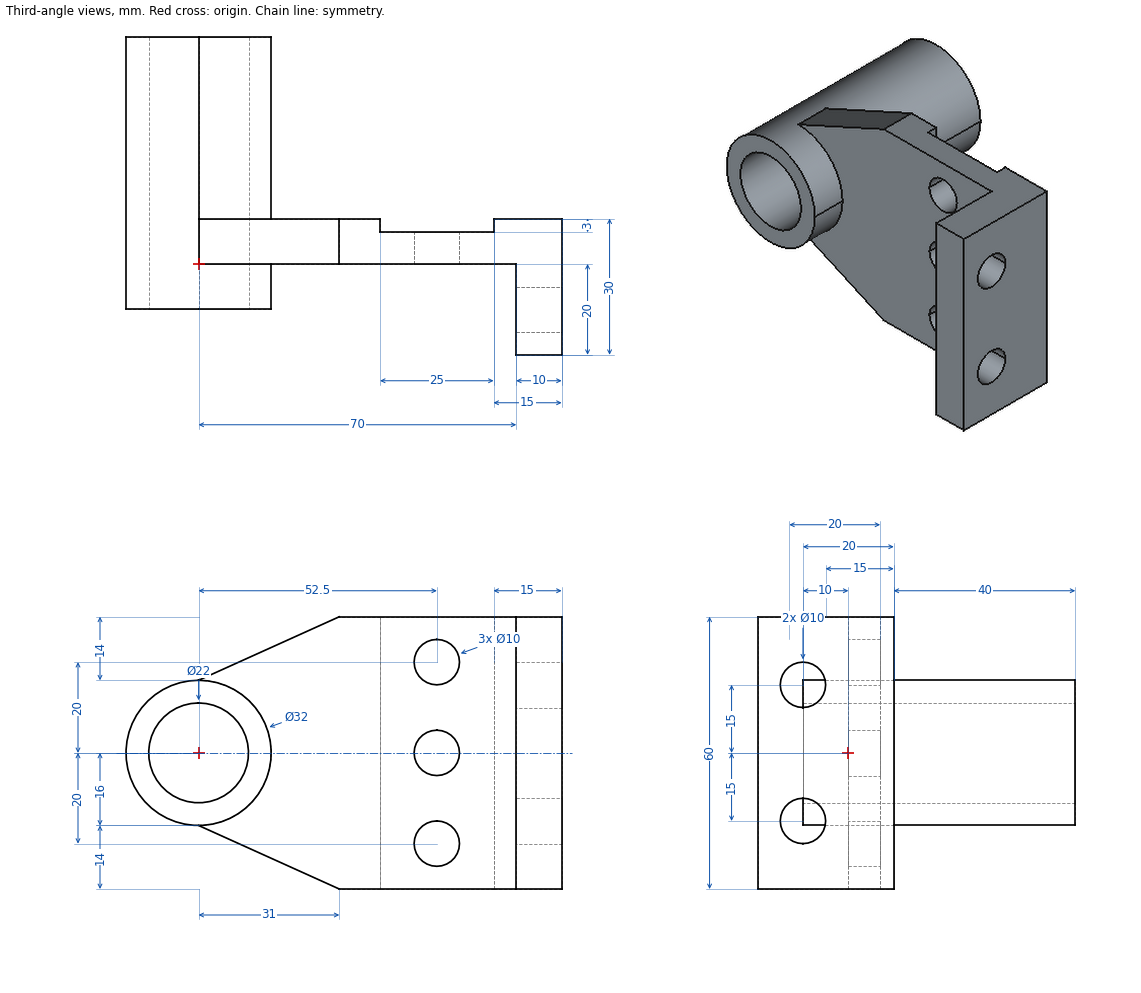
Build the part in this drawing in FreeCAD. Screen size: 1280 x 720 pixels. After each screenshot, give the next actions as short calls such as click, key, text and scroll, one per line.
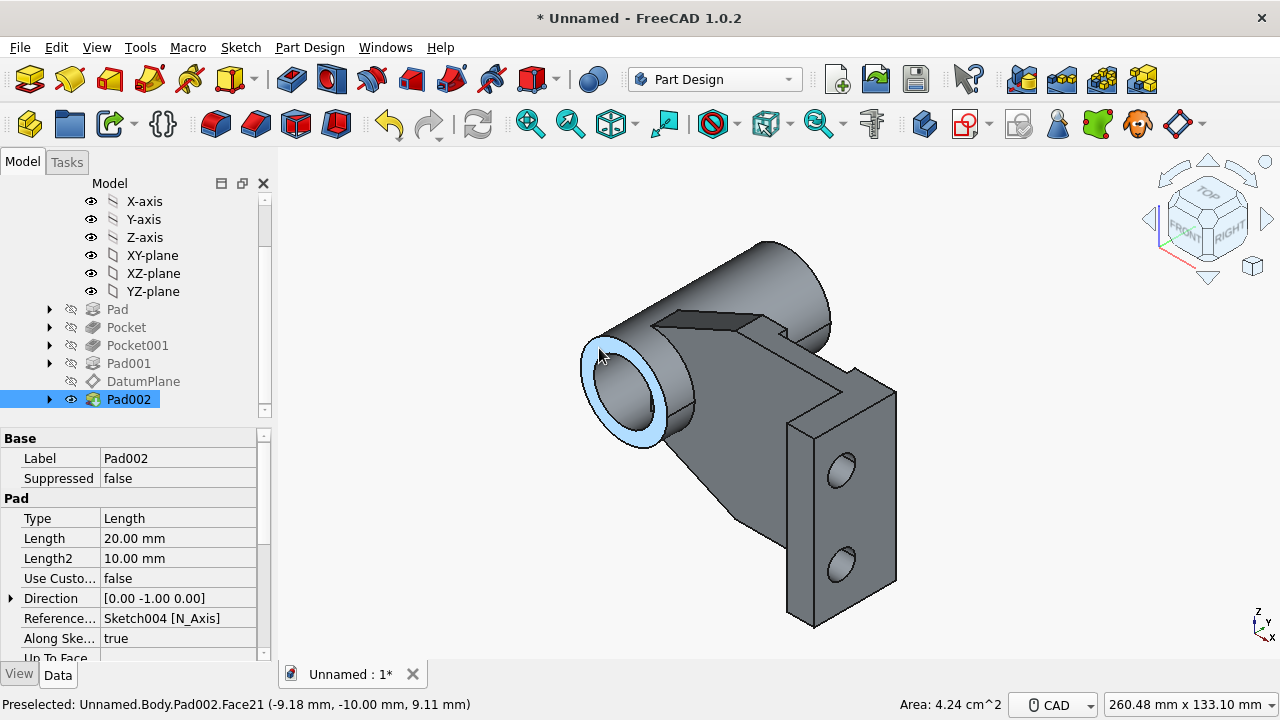
click(966, 124)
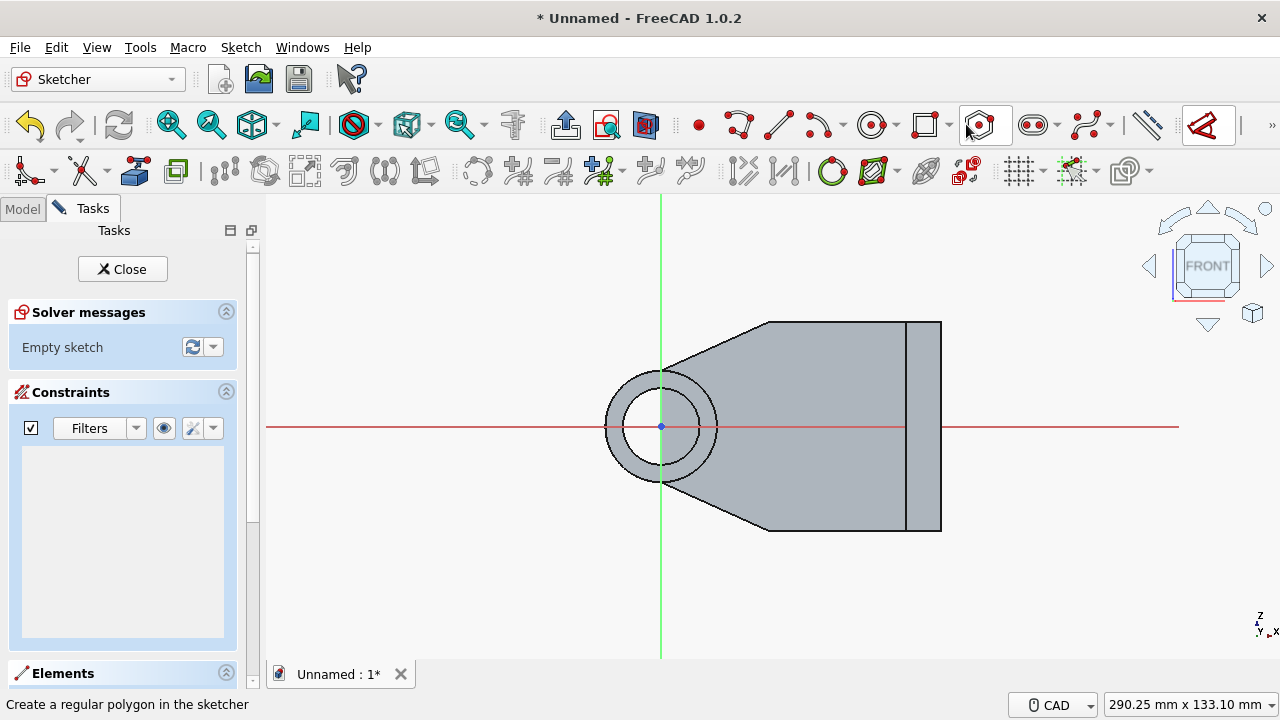
scroll(647, 426, up, 7)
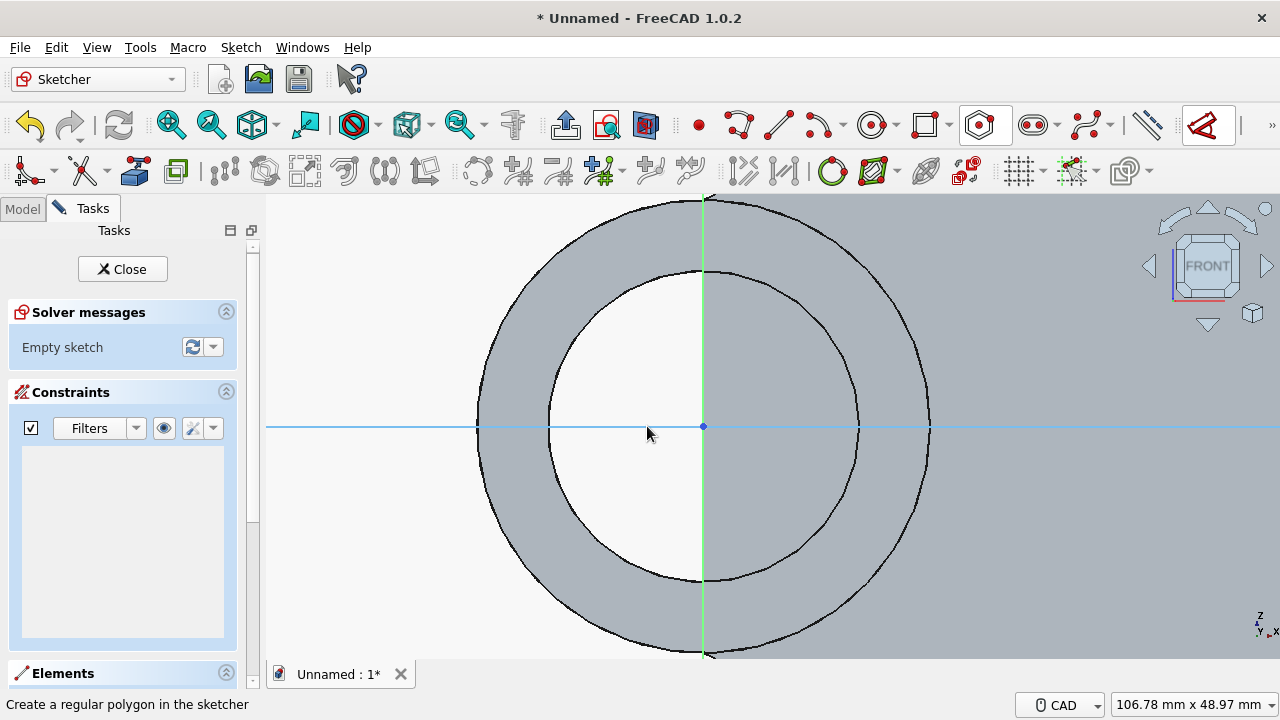
click(872, 126)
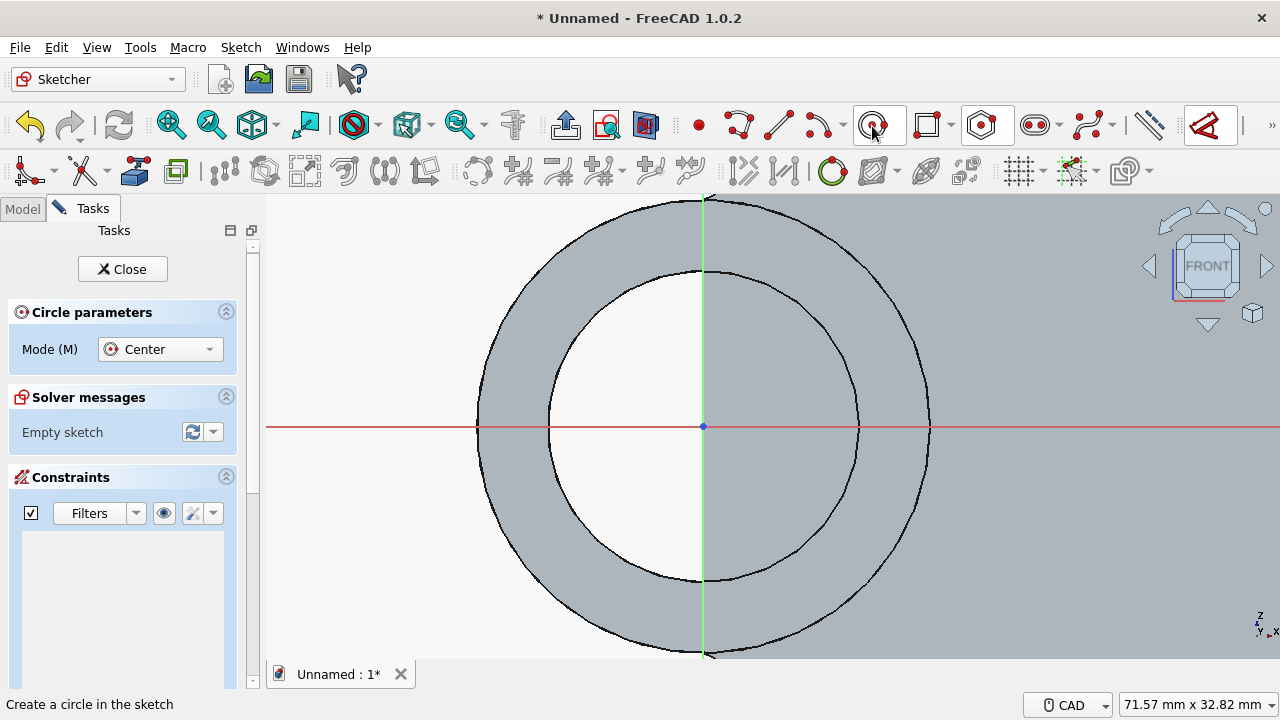
click(703, 426)
move(814, 316)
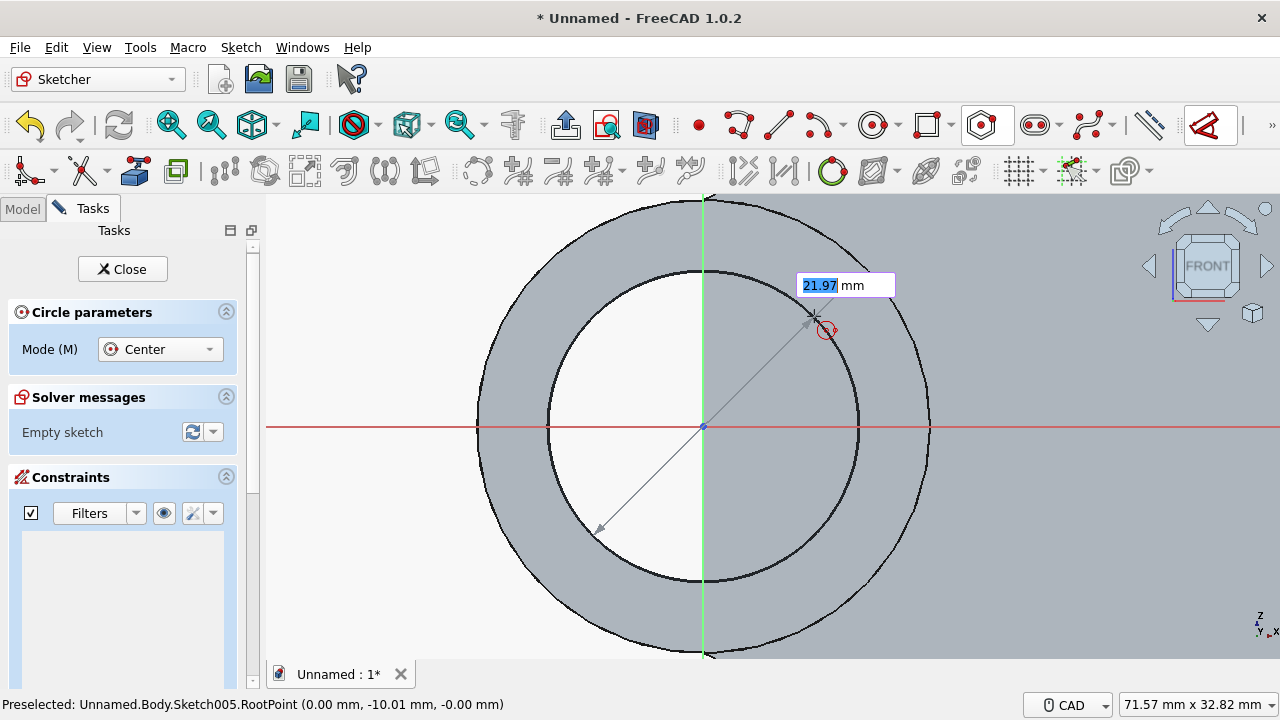
text(22)
key(Return)
key(Escape)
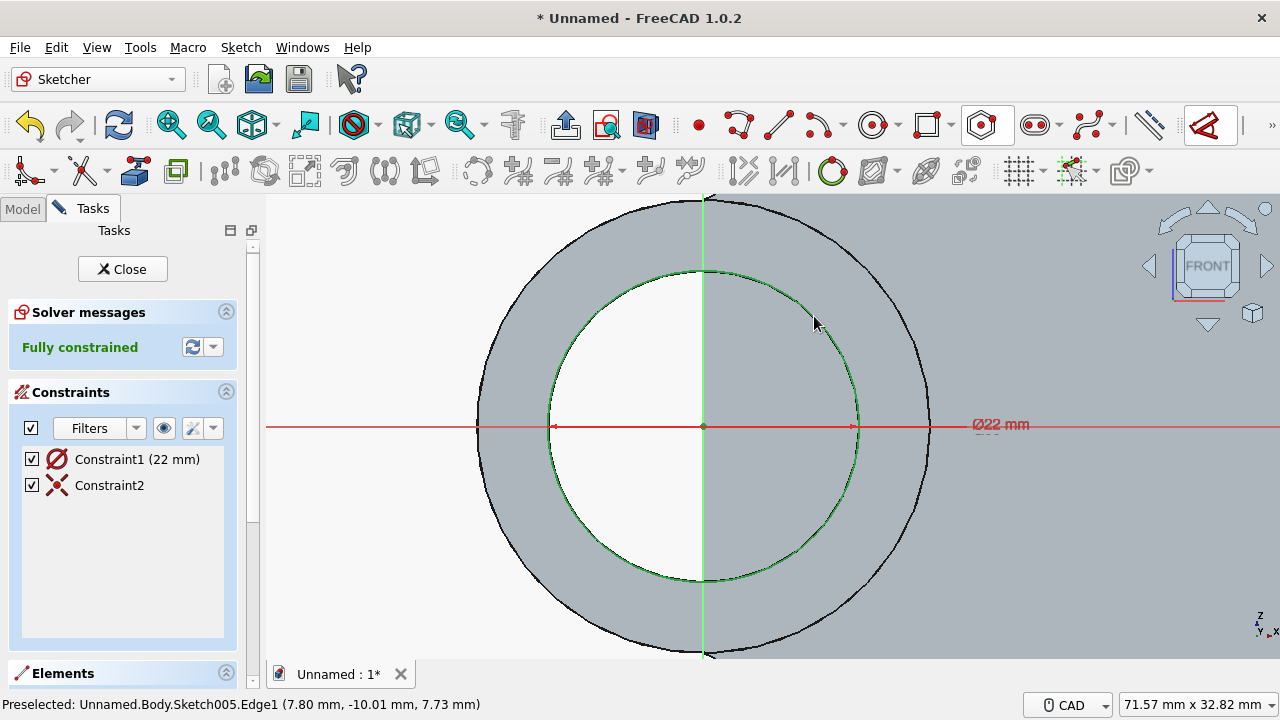
click(123, 269)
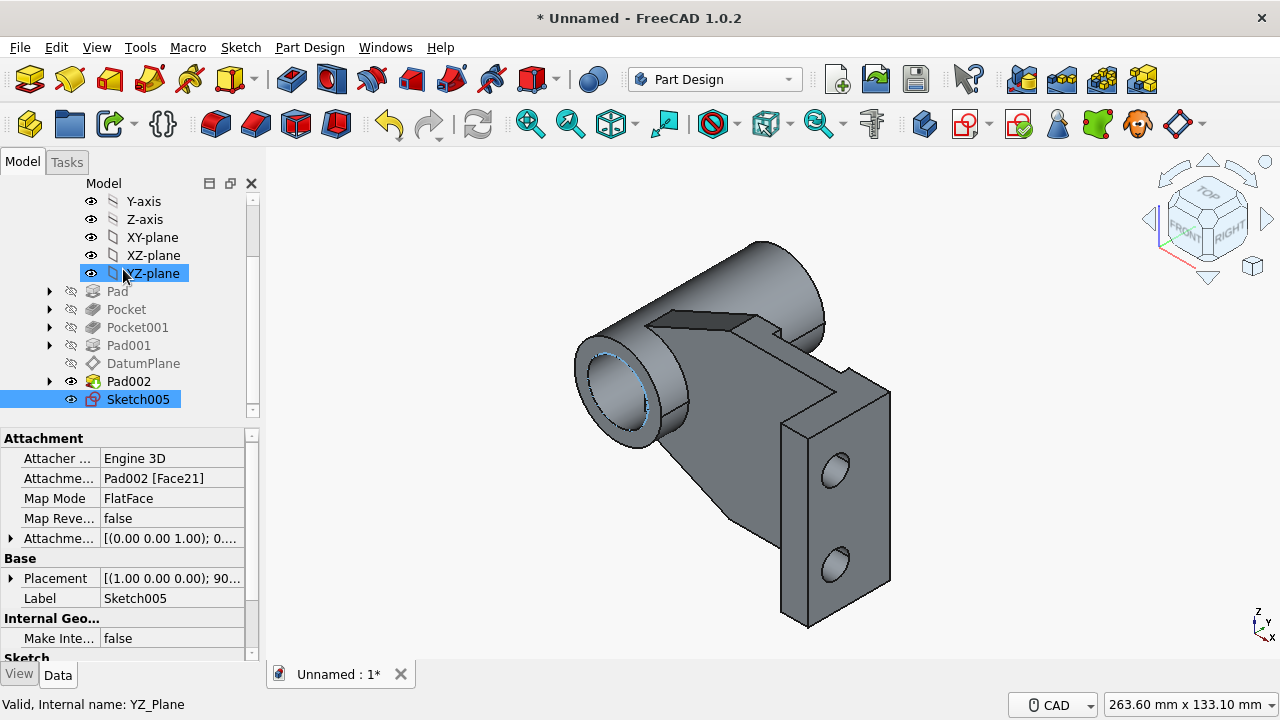
click(292, 80)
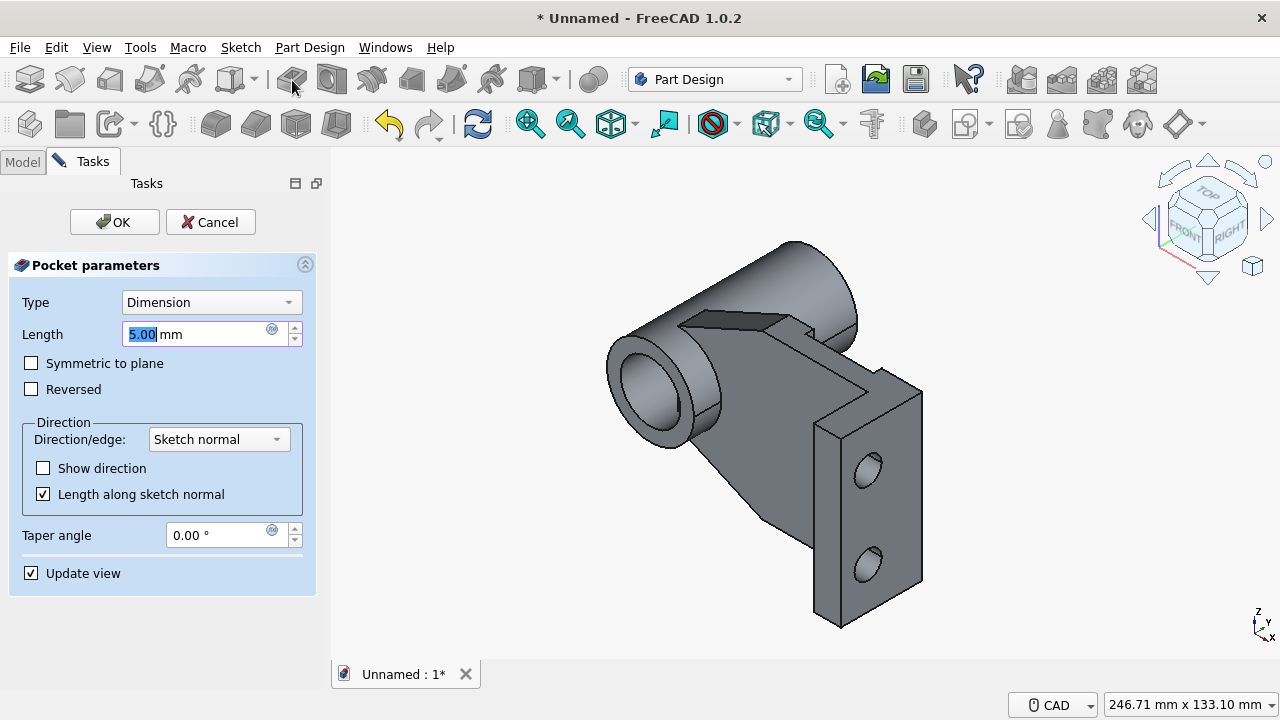
text(20)
key(Tab)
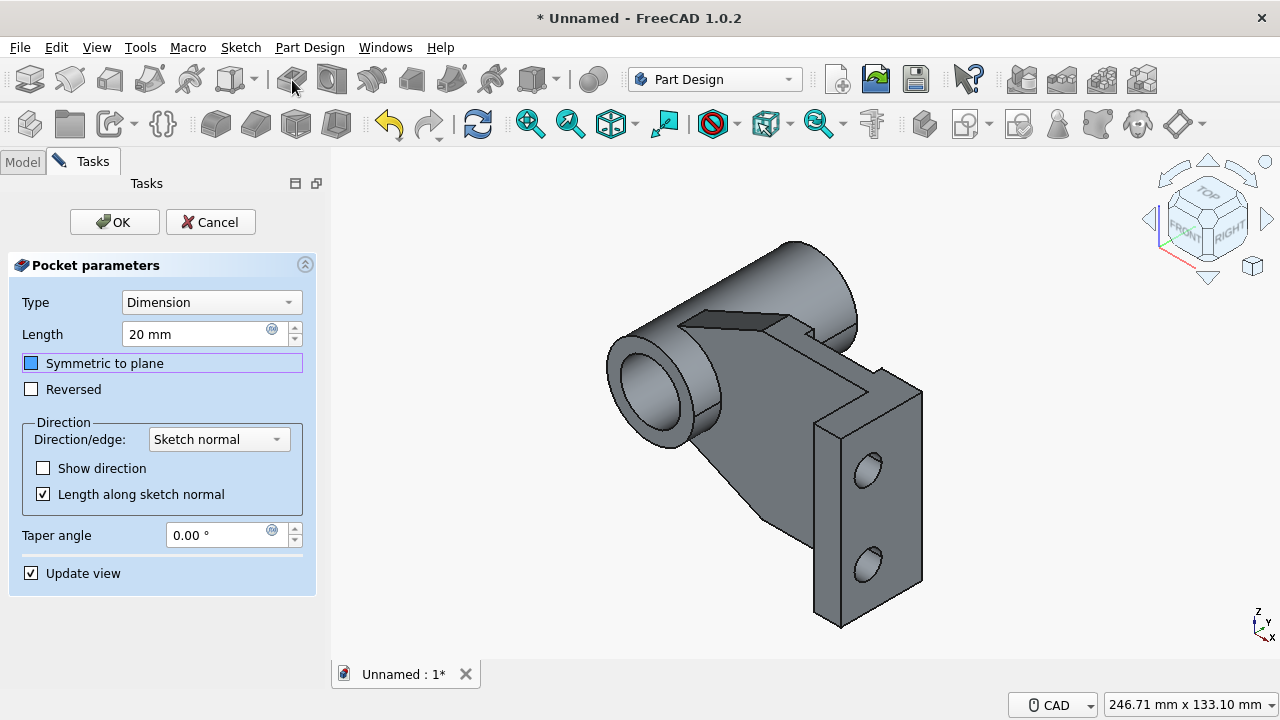
click(115, 222)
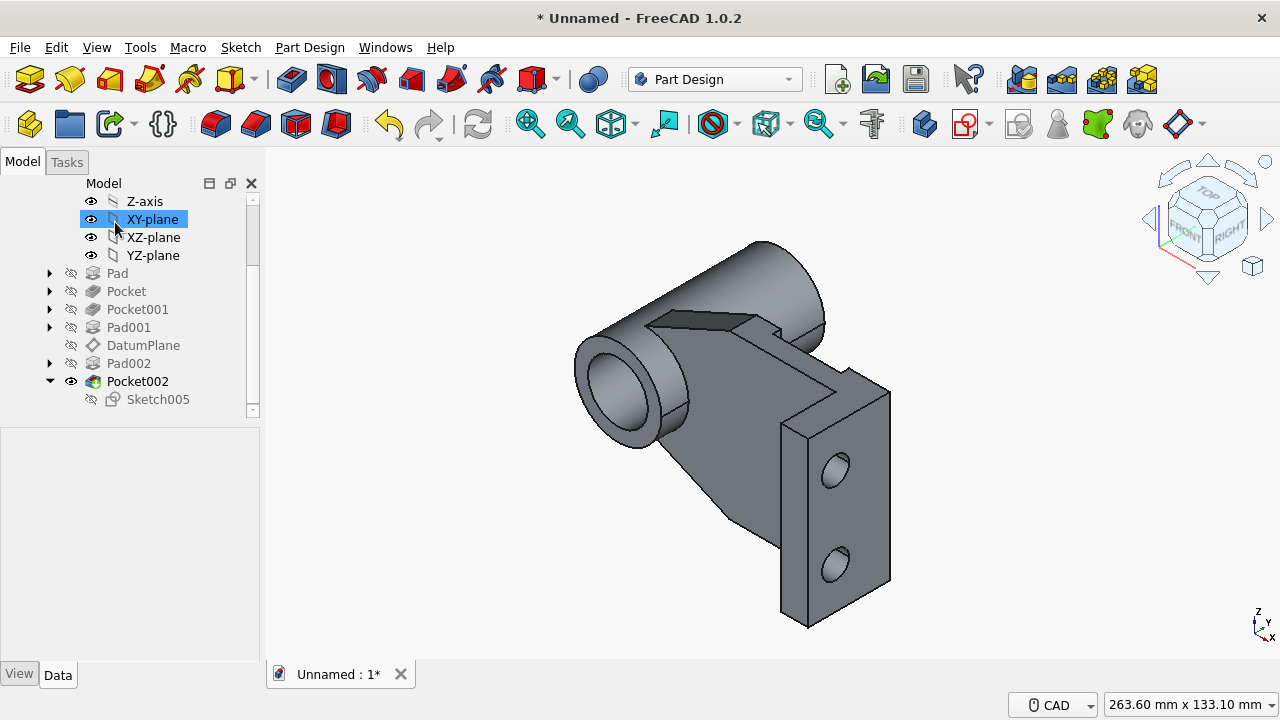
key(4)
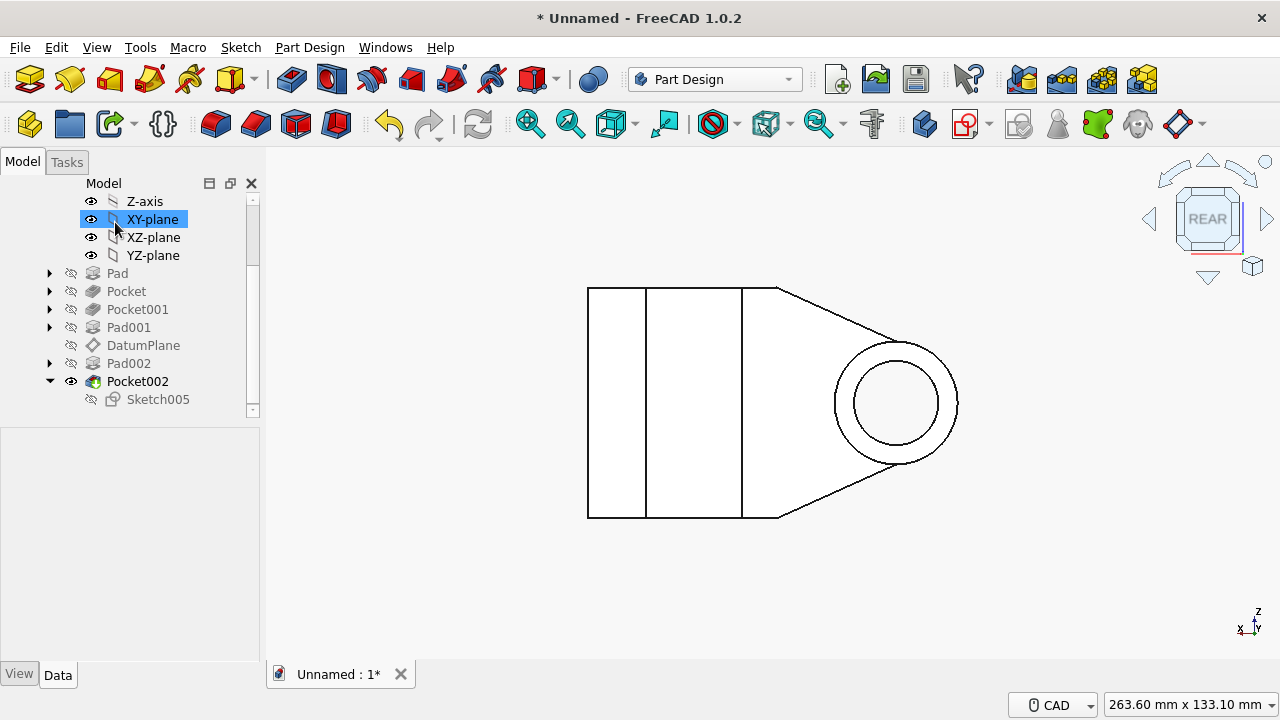
click(532, 124)